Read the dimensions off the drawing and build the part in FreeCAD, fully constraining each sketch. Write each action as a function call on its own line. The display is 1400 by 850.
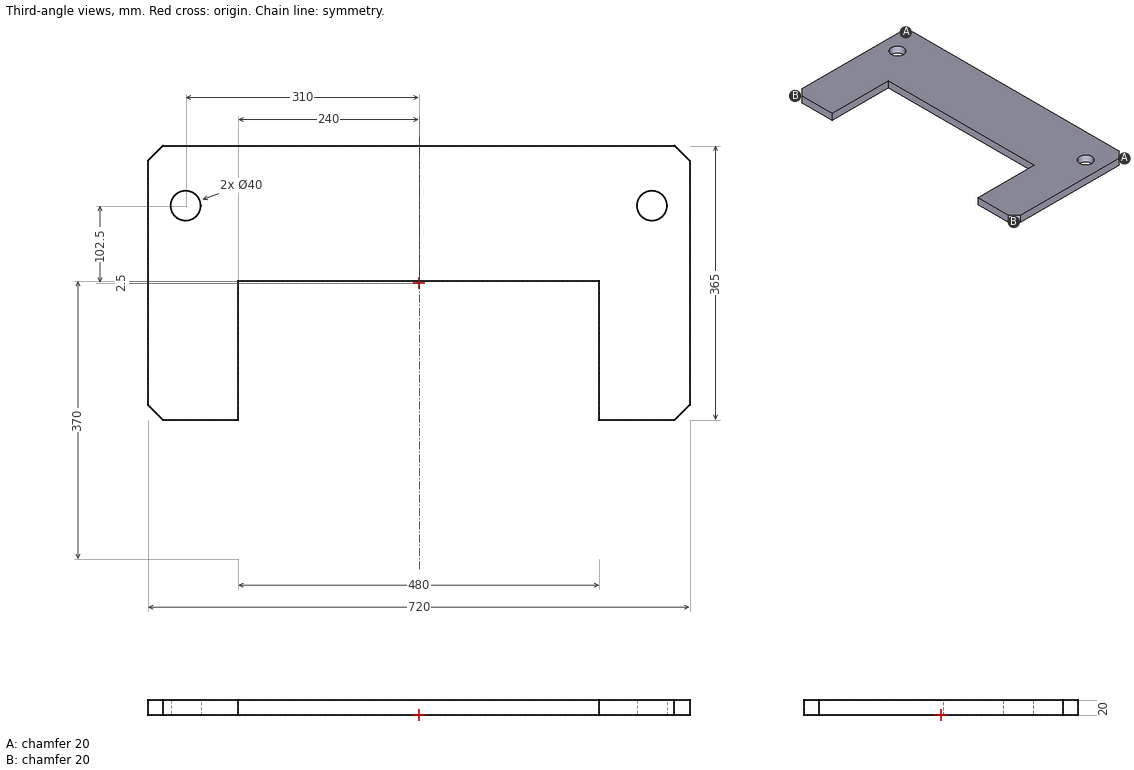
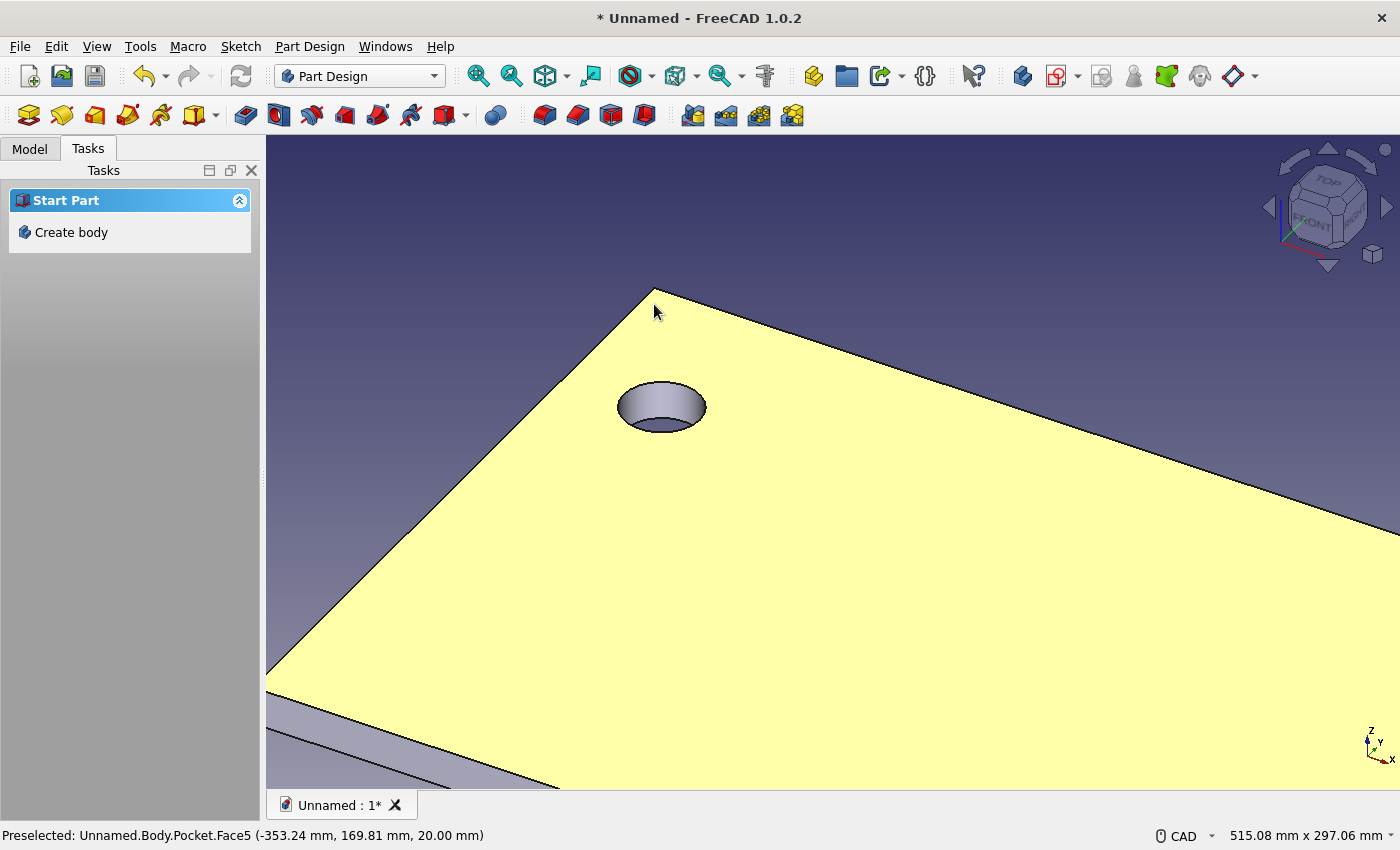
click(479, 76)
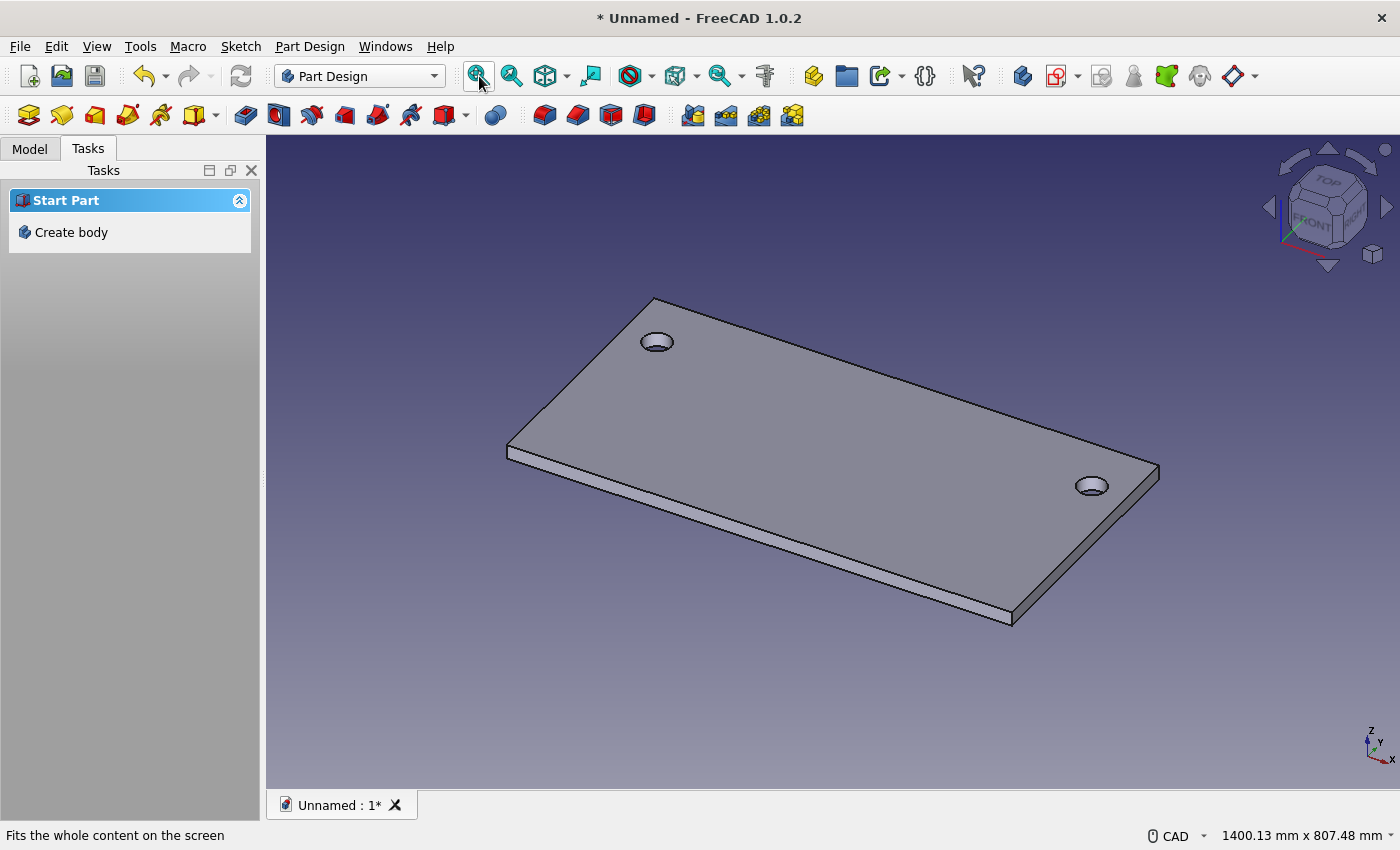
key(0)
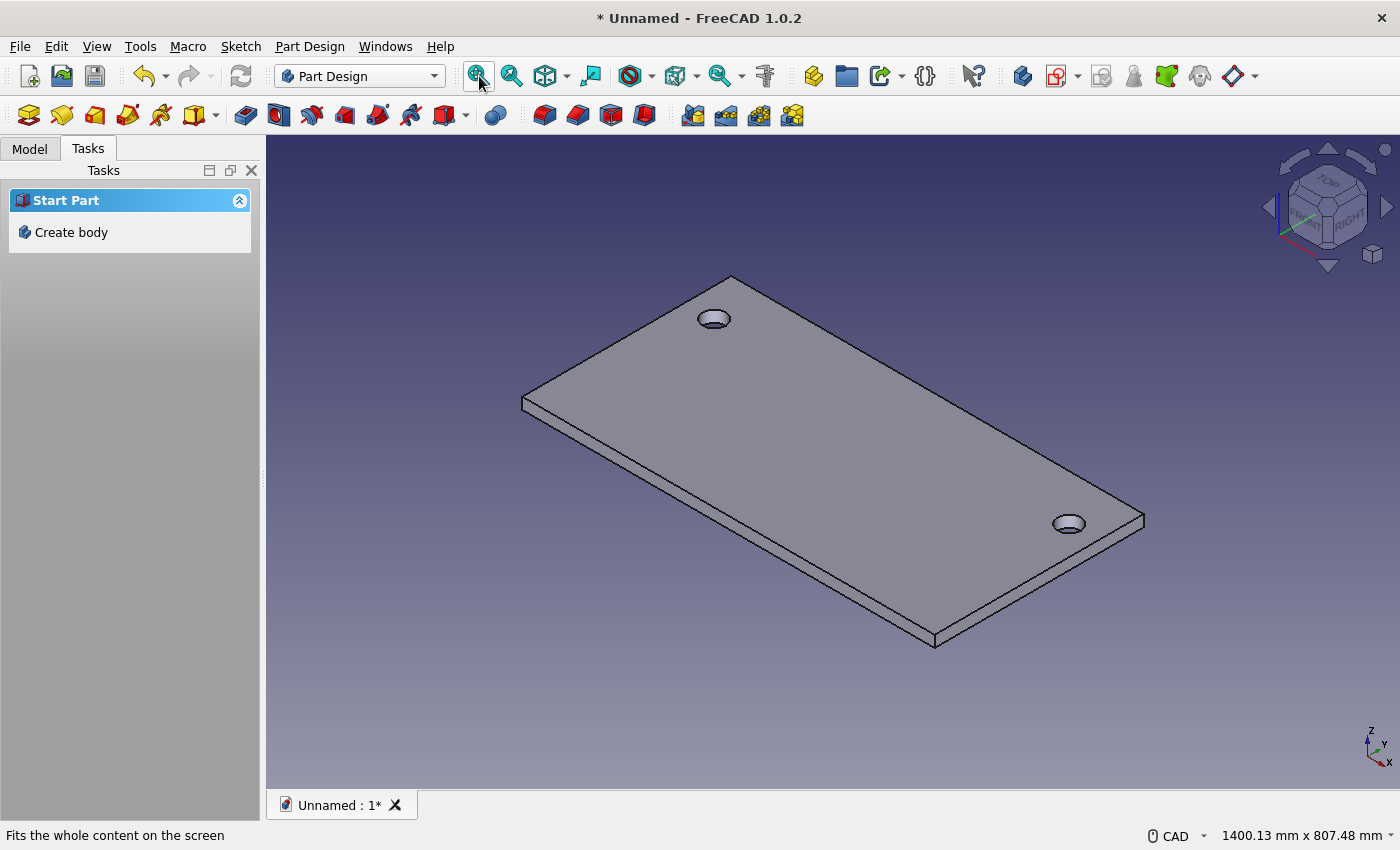
scroll(731, 282, up, 5)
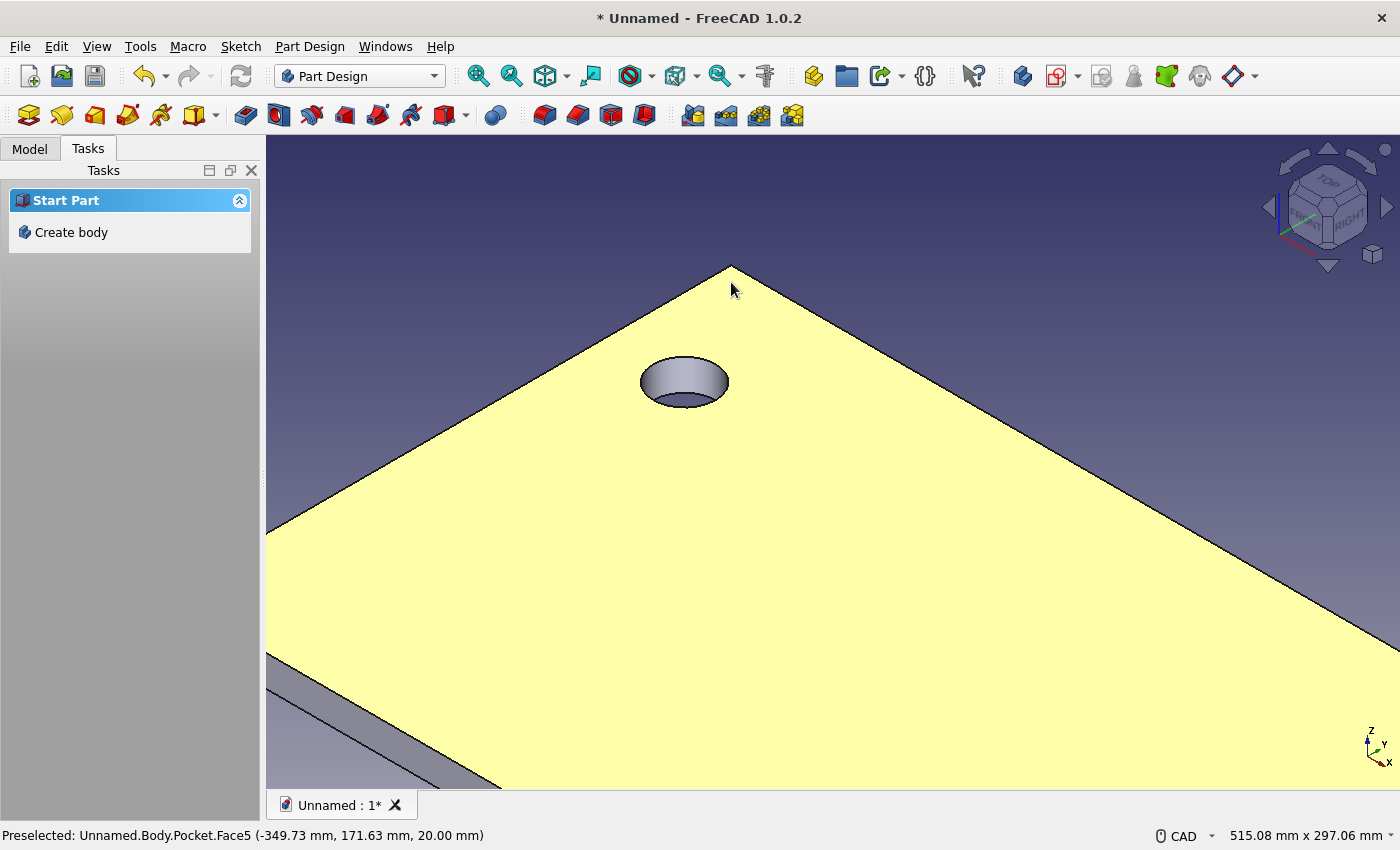
key(v)
key(f)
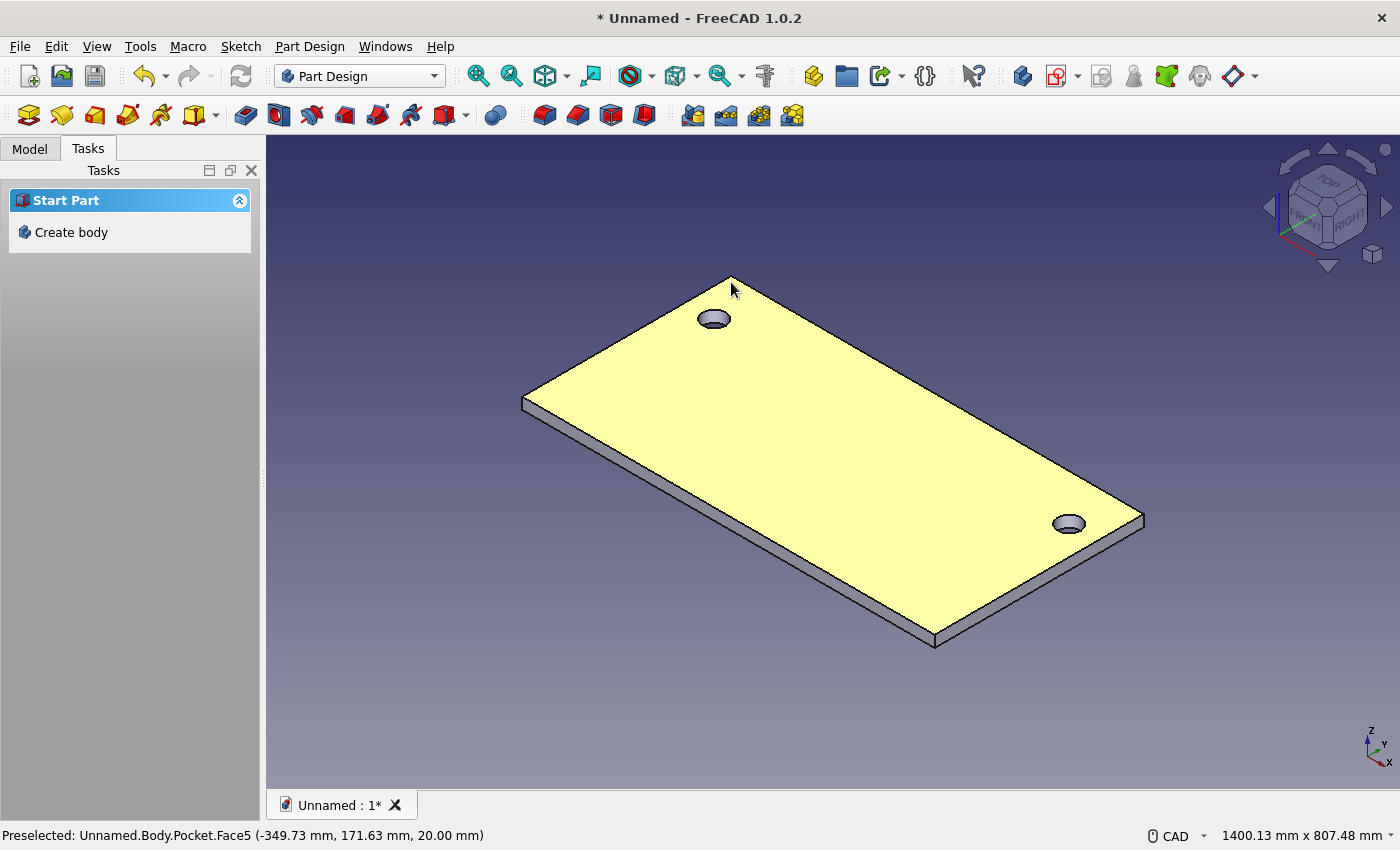
key(2)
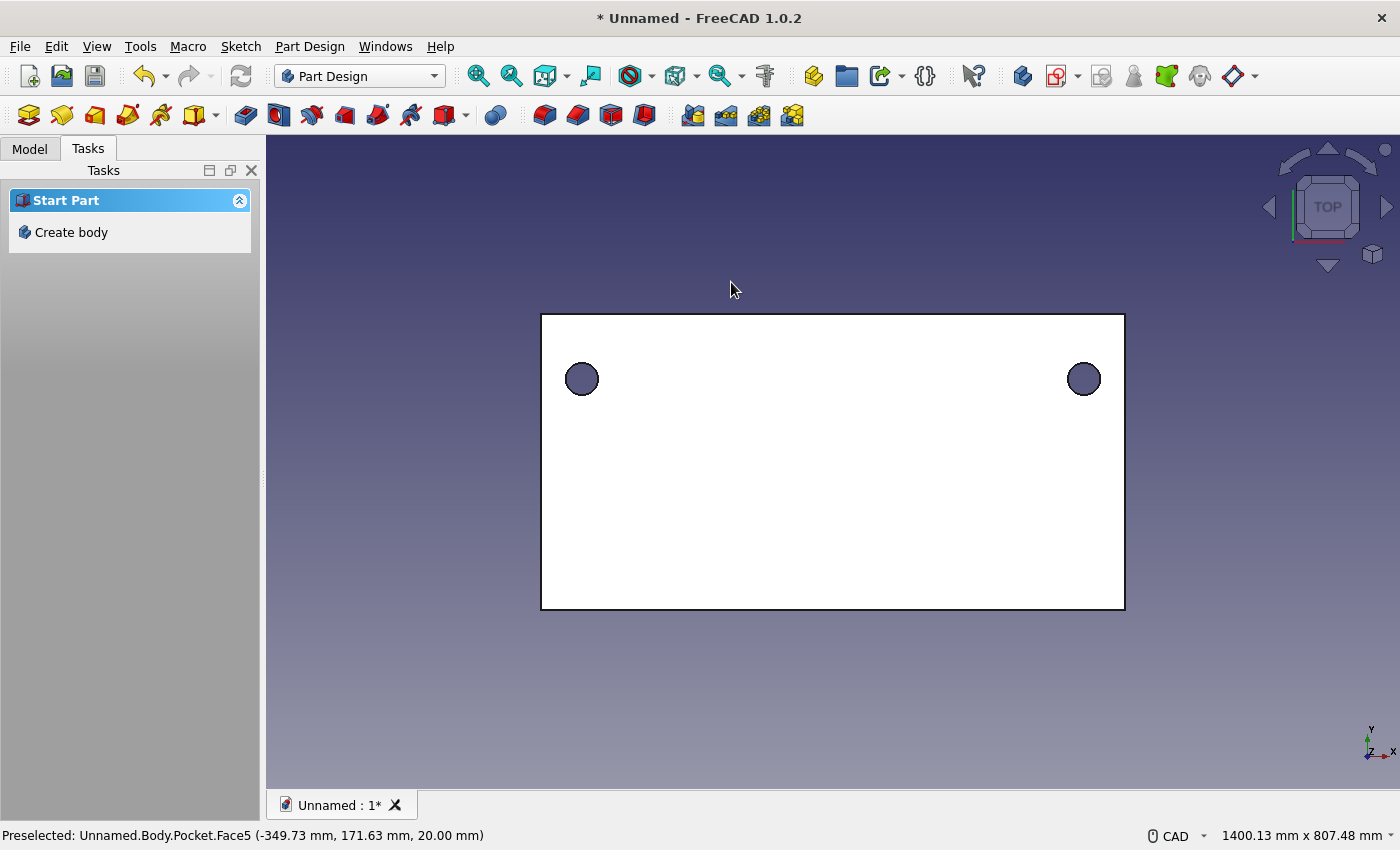
scroll(541, 313, up, 5)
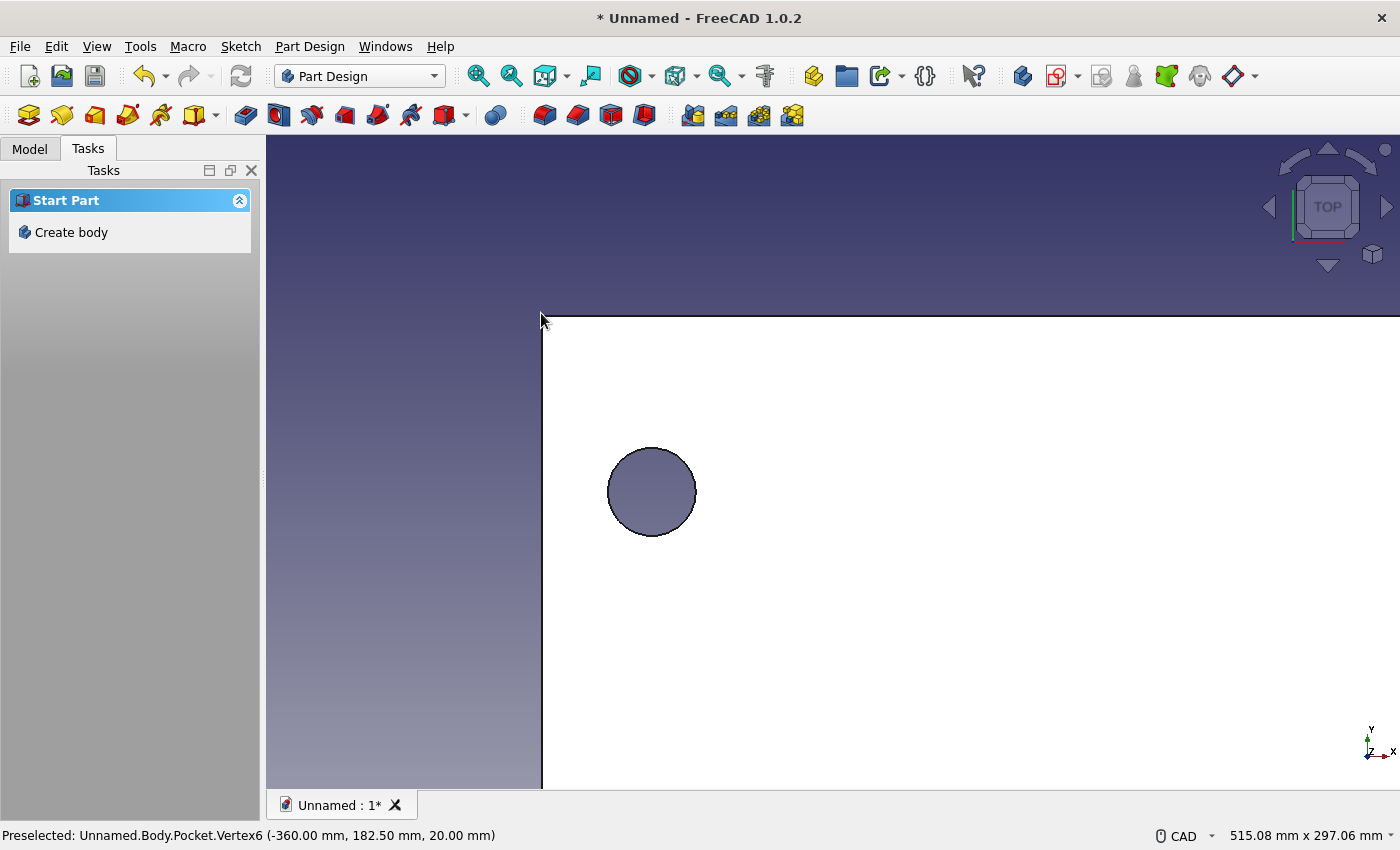
click(479, 76)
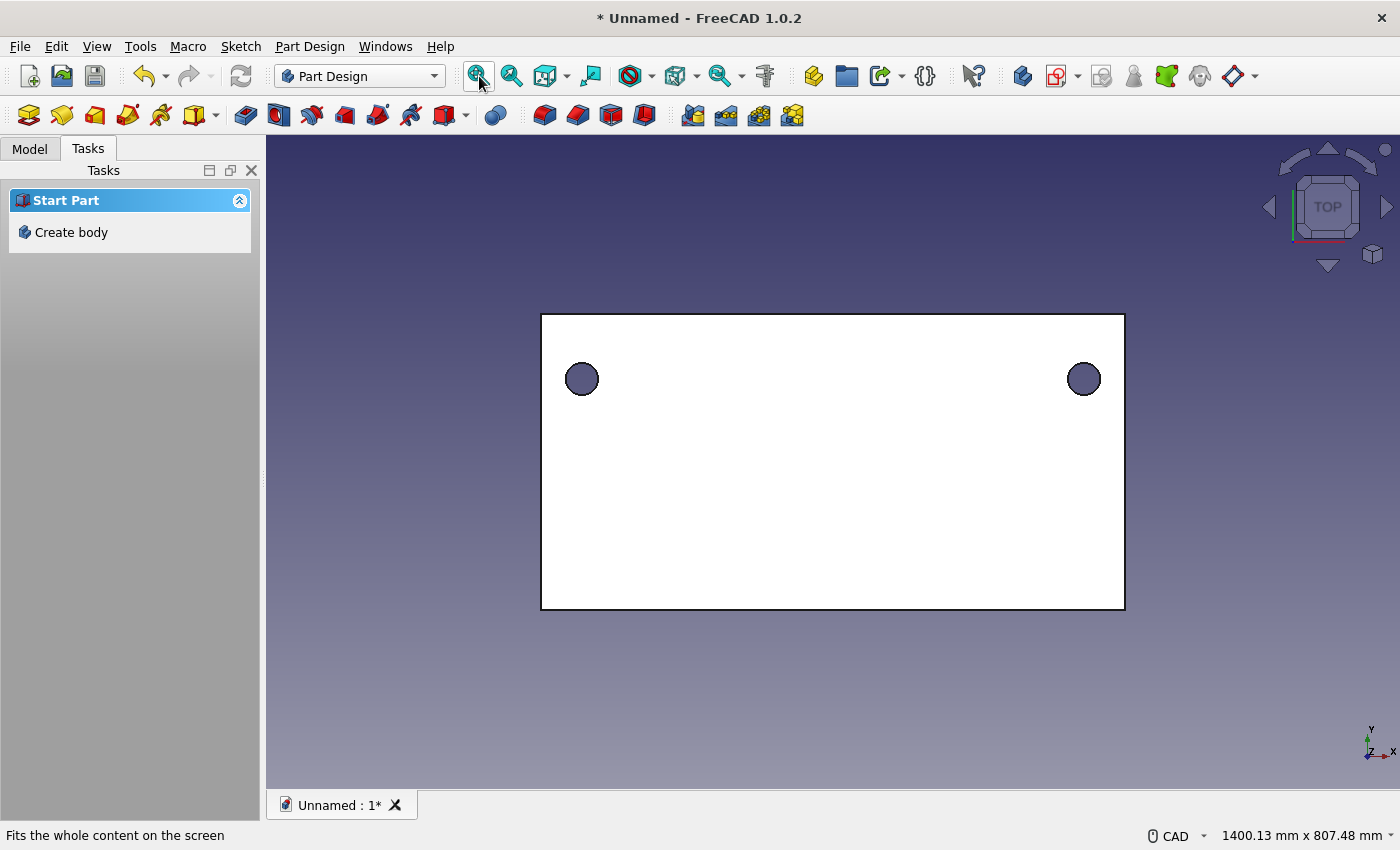
key(1)